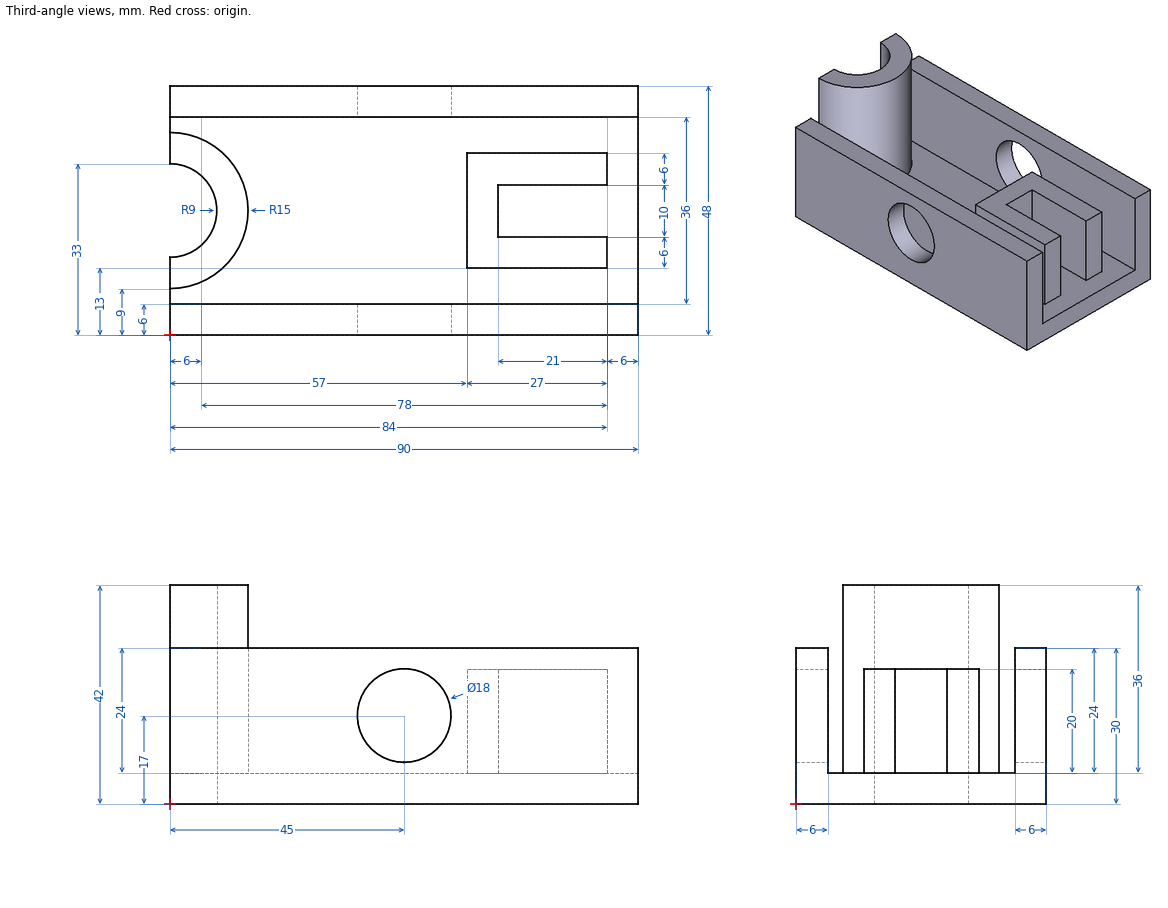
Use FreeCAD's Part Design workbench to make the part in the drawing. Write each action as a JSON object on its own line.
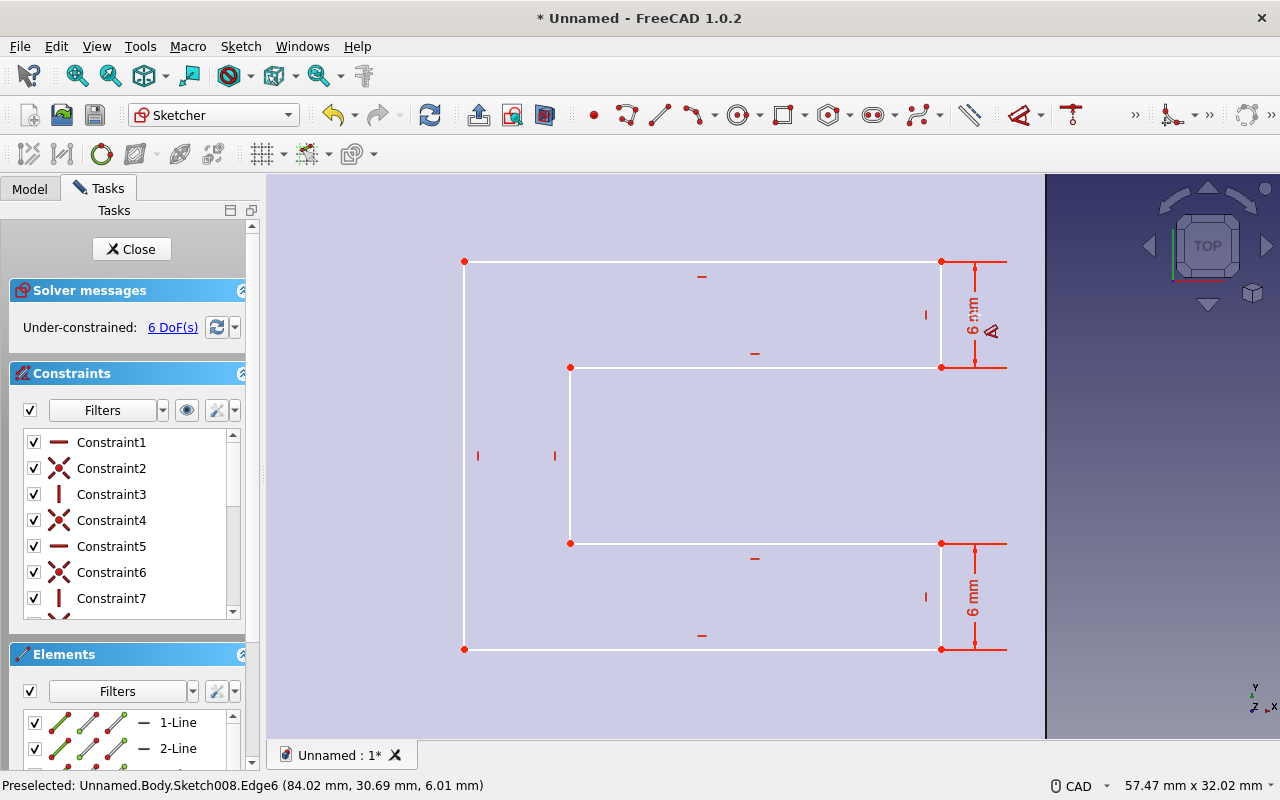
{"action": "left_click", "coordinate": [607, 650]}
{"action": "left_click", "coordinate": [702, 684]}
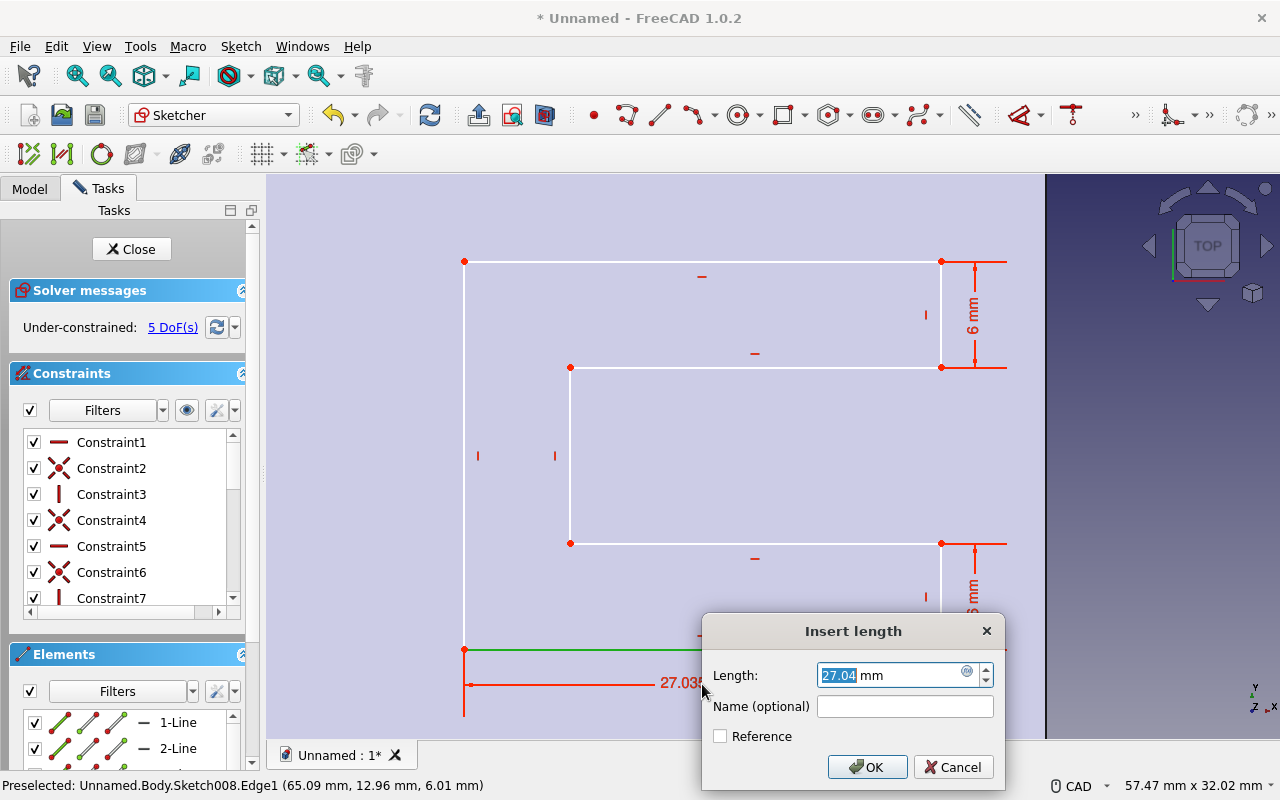
{"action": "type", "text": "27"}
{"action": "key", "text": "Return"}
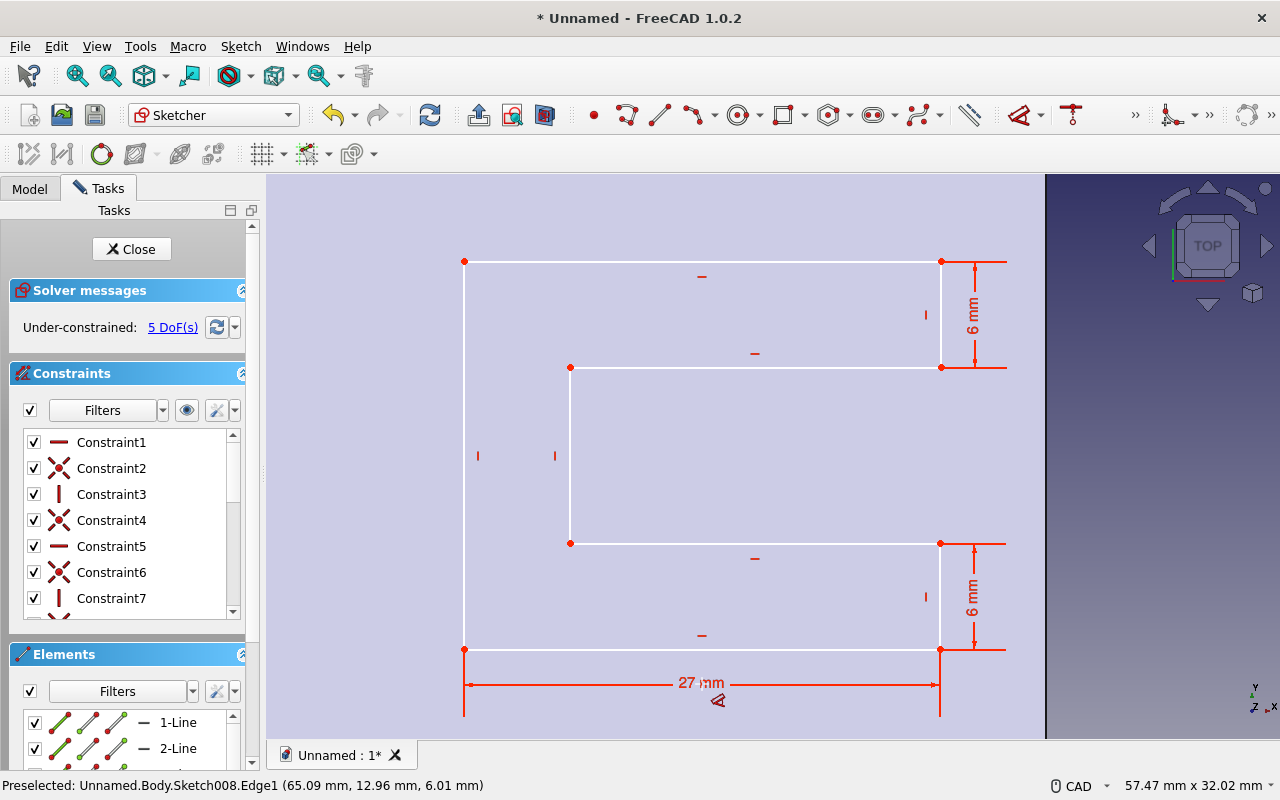
{"action": "left_click", "coordinate": [829, 544]}
{"action": "left_click", "coordinate": [755, 578]}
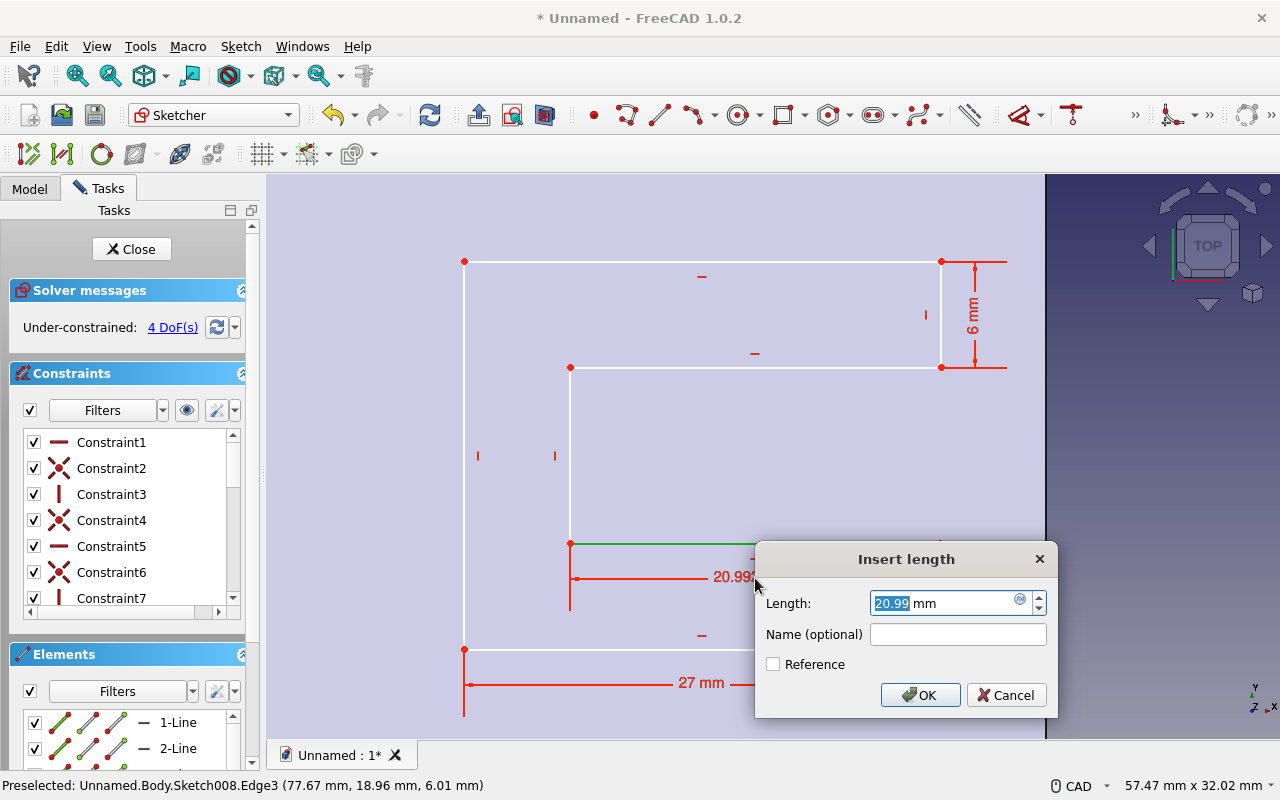
{"action": "type", "text": "21"}
{"action": "key", "text": "Return"}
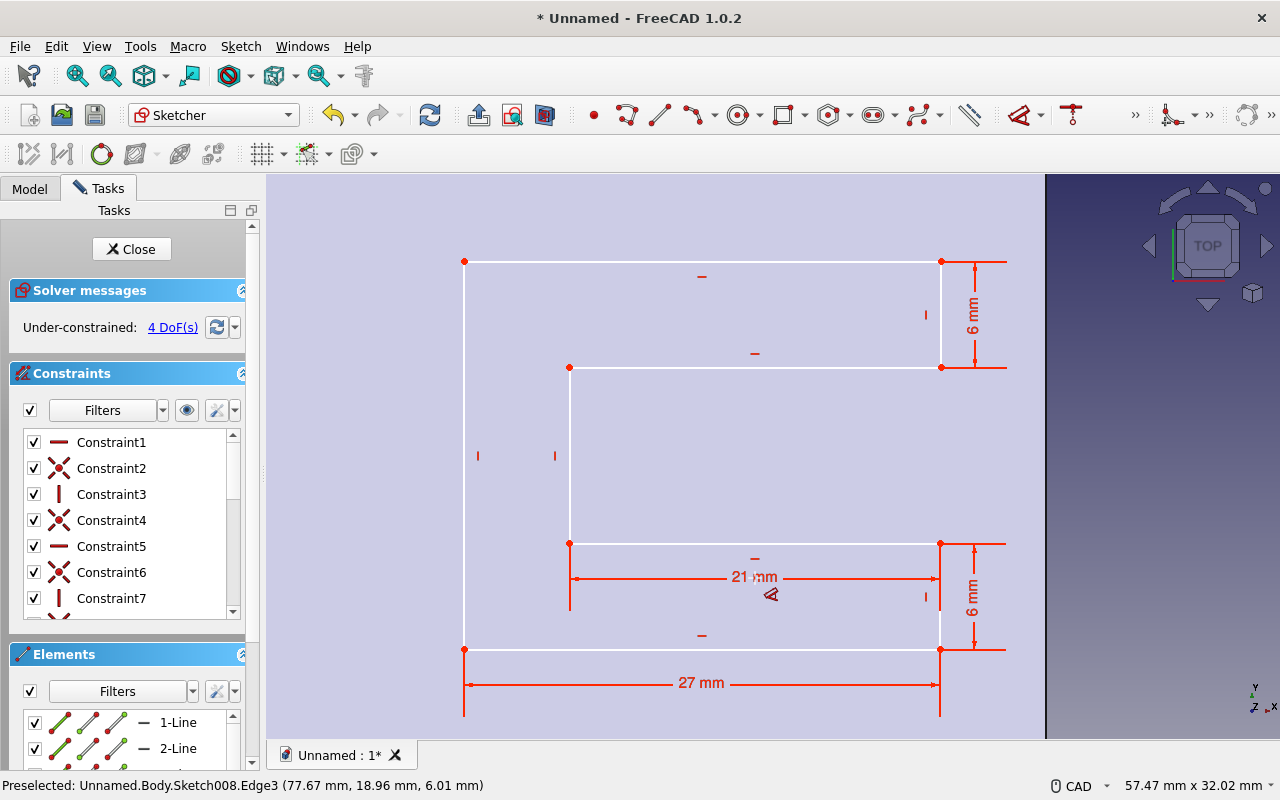
{"action": "left_click", "coordinate": [570, 491]}
{"action": "left_click", "coordinate": [536, 456]}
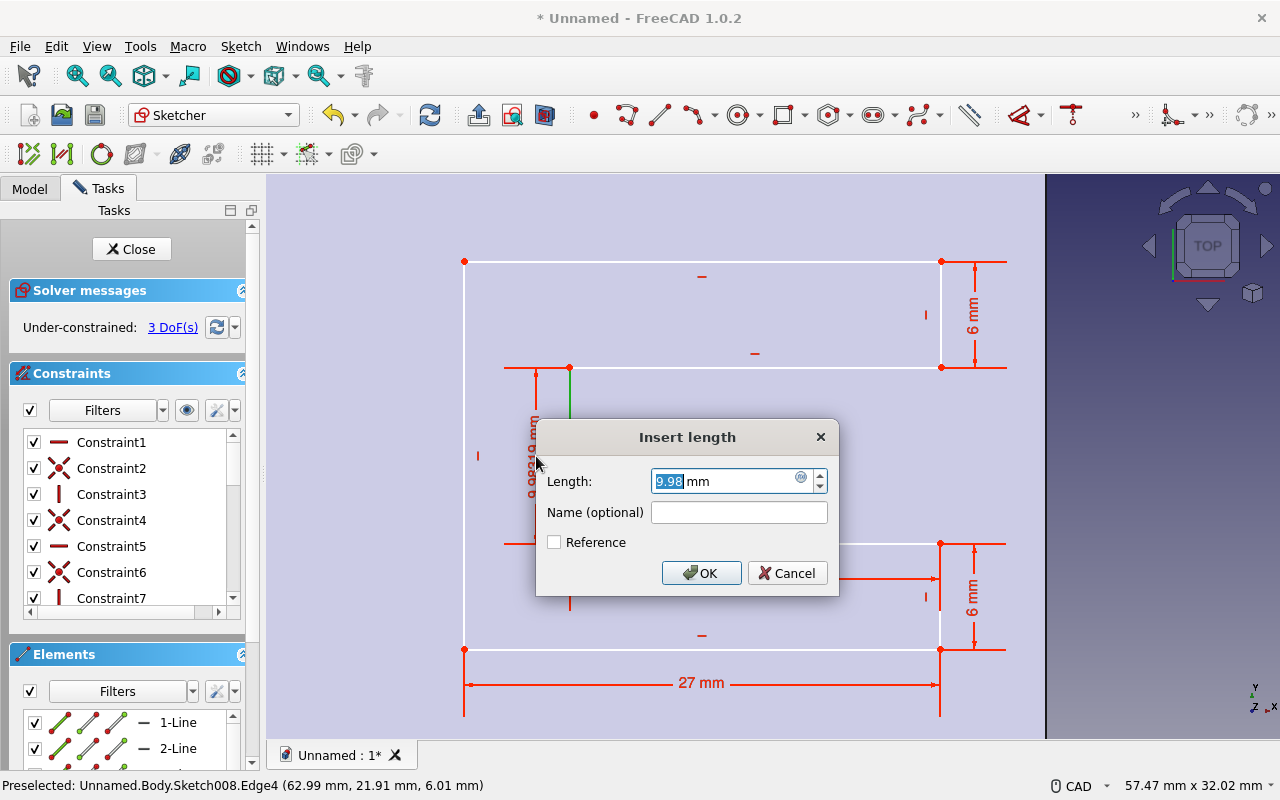
{"action": "type", "text": "10"}
{"action": "key", "text": "Return"}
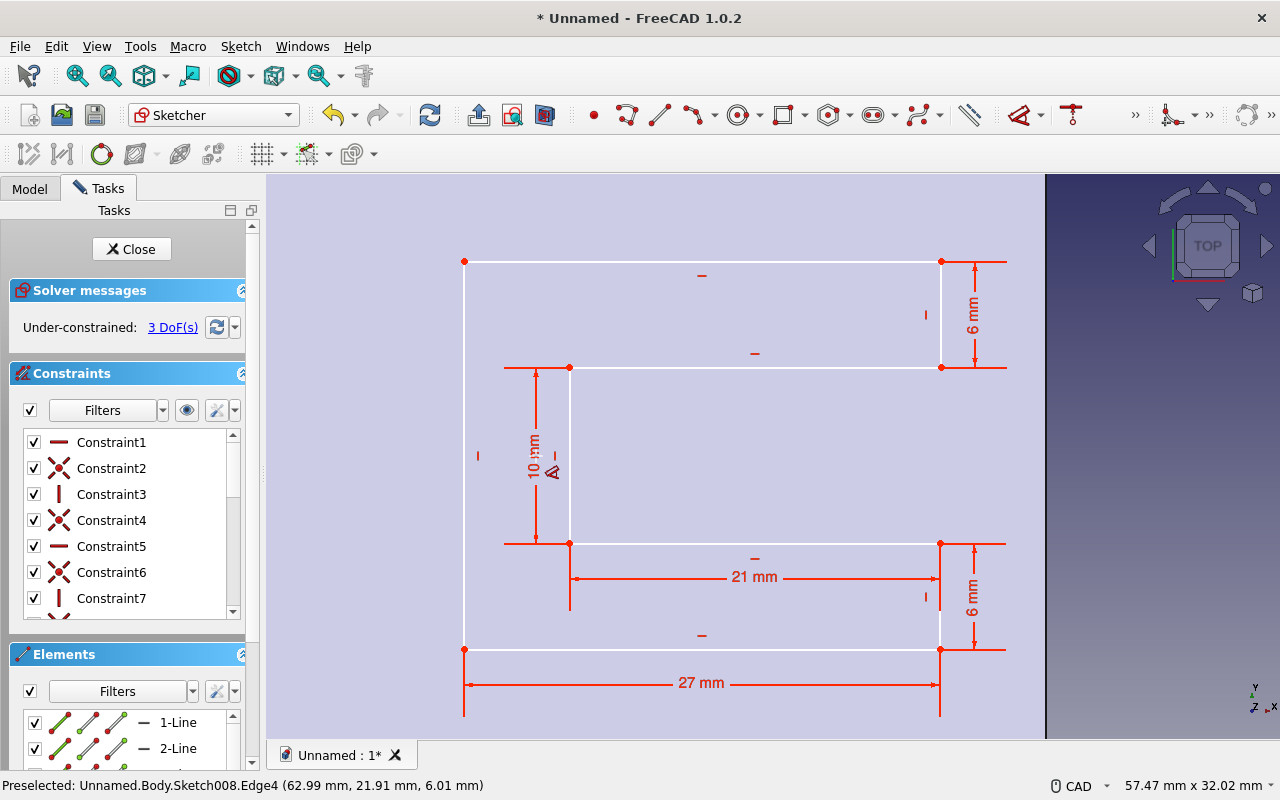
{"action": "left_click", "coordinate": [681, 368]}
{"action": "left_click", "coordinate": [755, 334]}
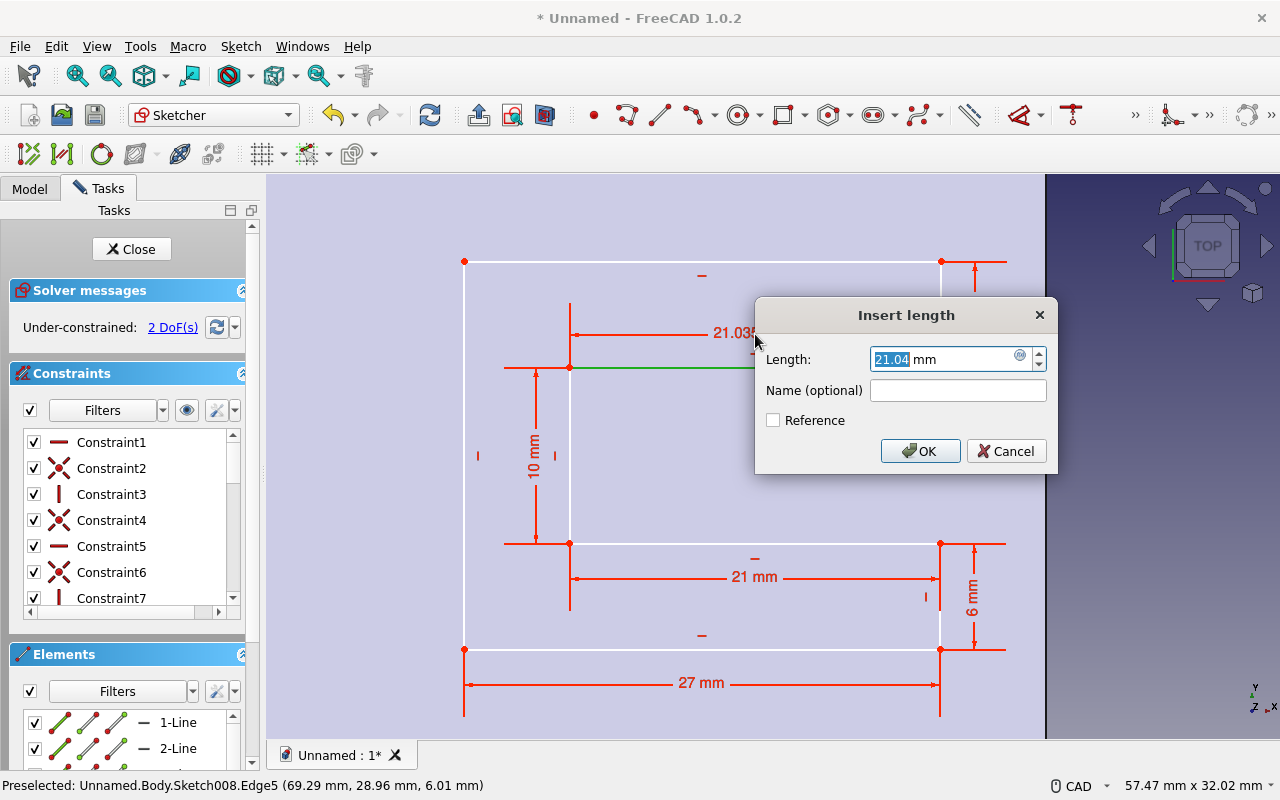
{"action": "type", "text": "21"}
{"action": "key", "text": "Return"}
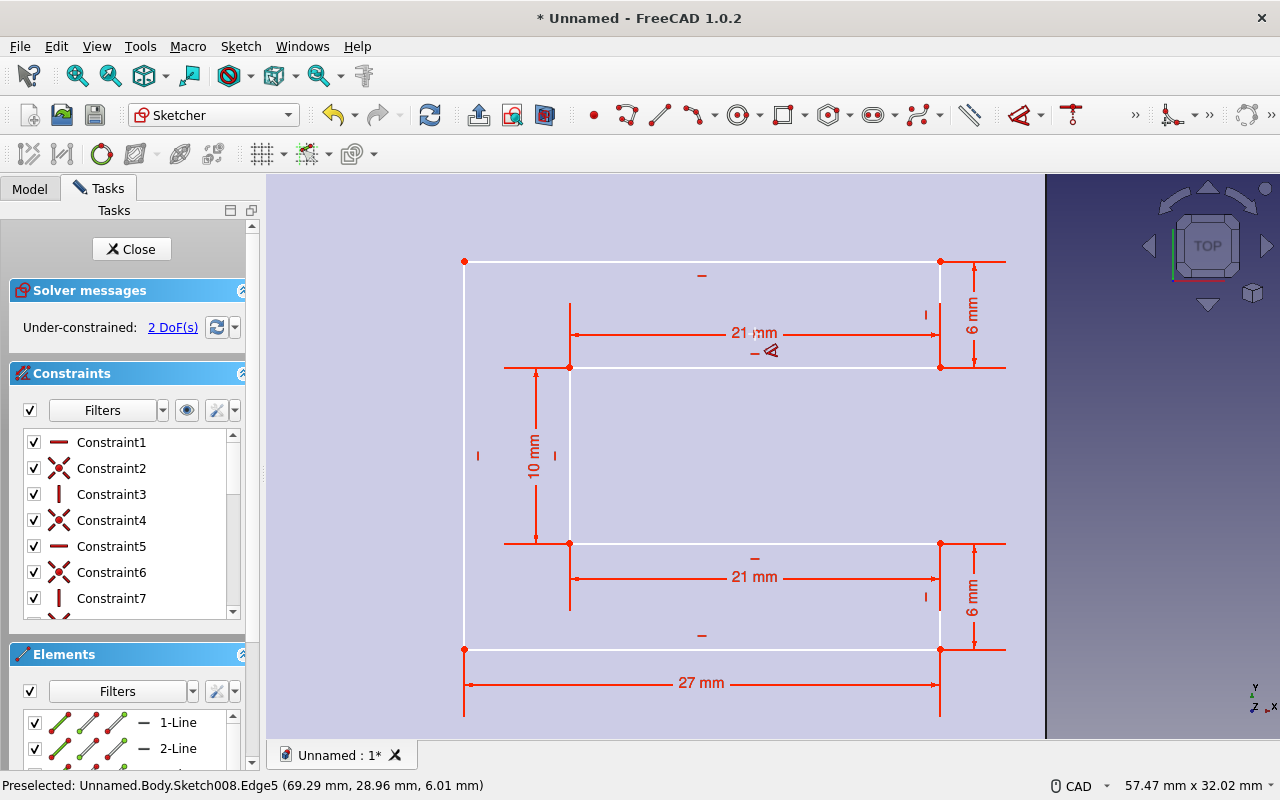
{"action": "left_click", "coordinate": [464, 650]}
{"action": "left_click", "coordinate": [379, 616]}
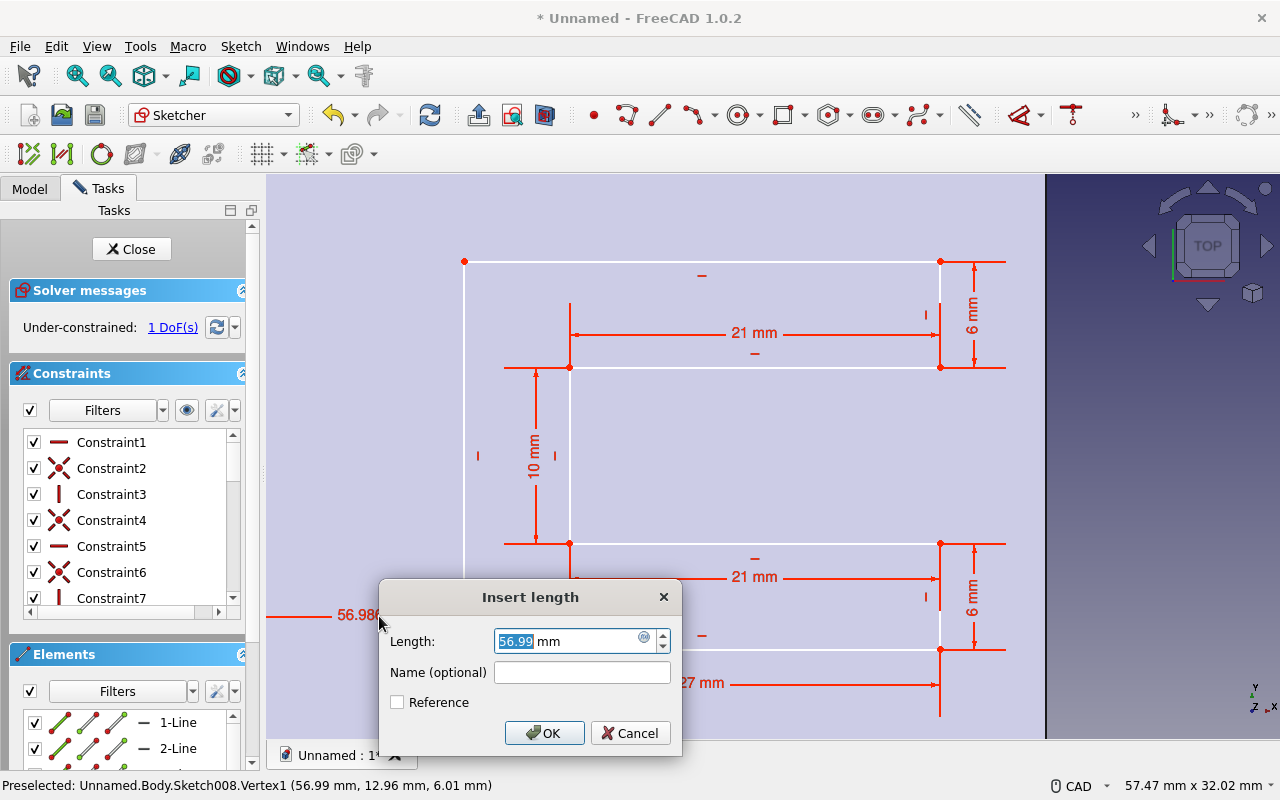
{"action": "type", "text": "57"}
{"action": "key", "text": "Return"}